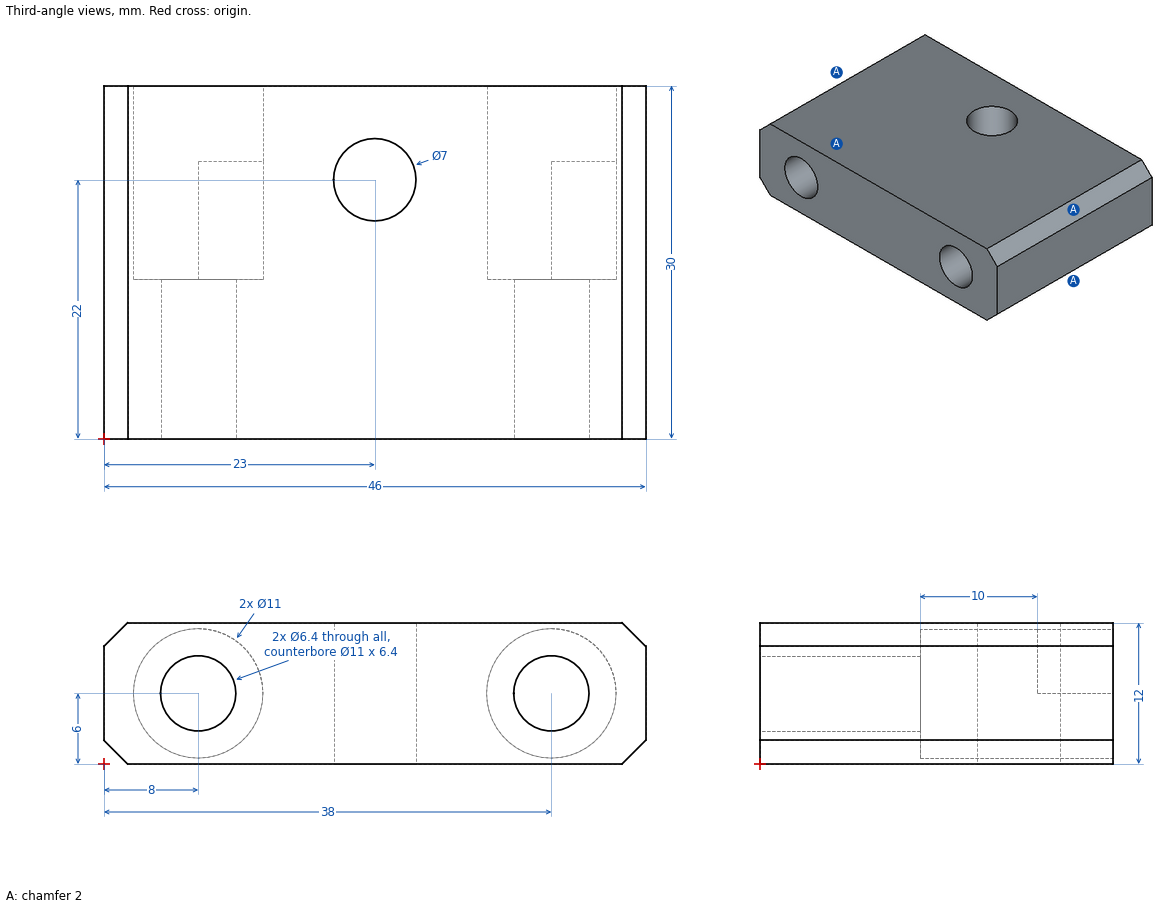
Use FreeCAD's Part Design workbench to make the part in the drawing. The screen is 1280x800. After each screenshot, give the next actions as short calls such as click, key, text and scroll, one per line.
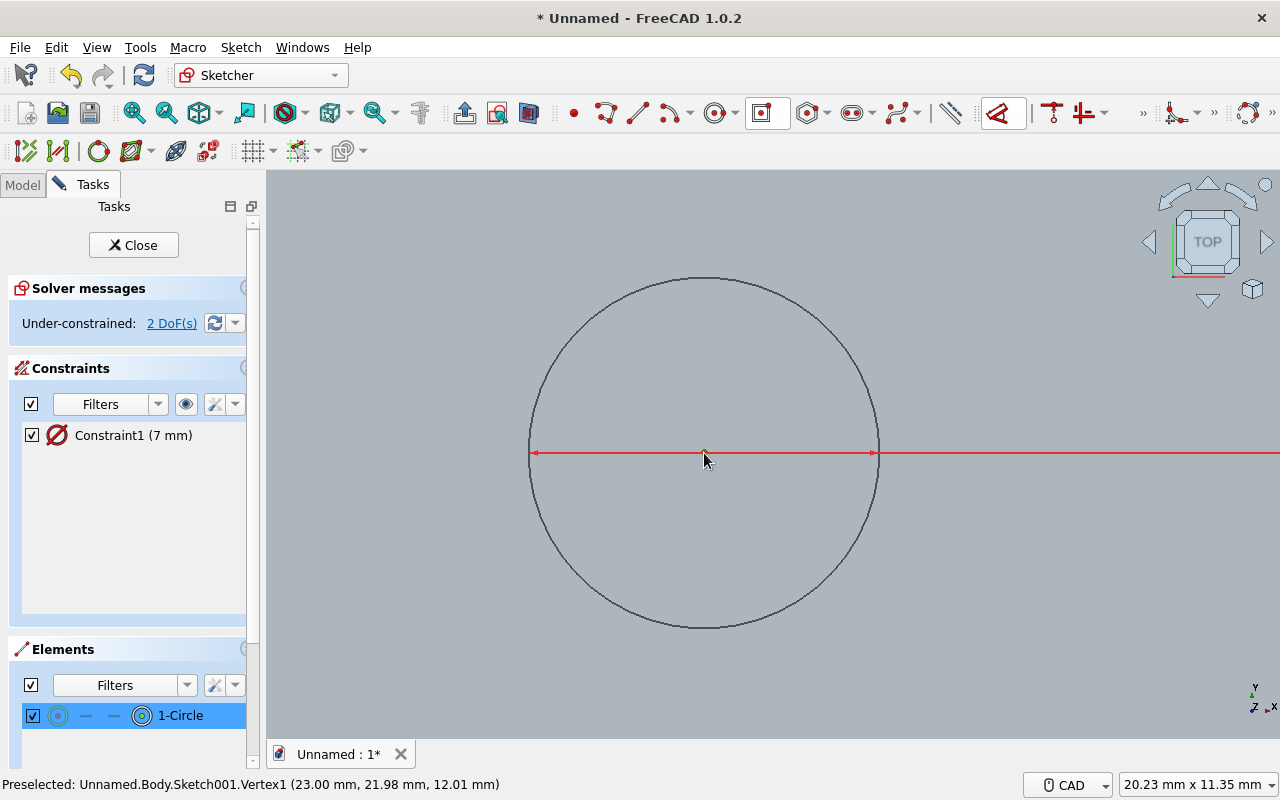
key(l)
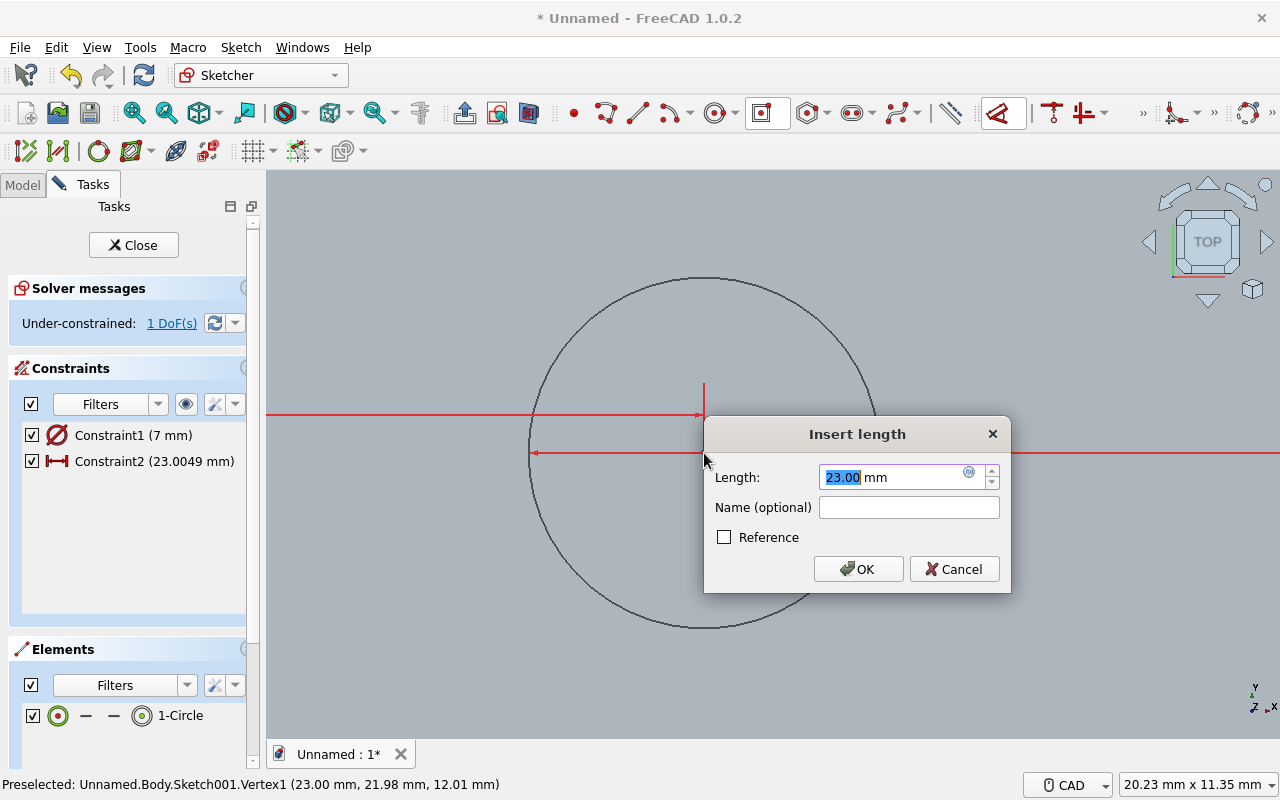
text(23)
key(Return)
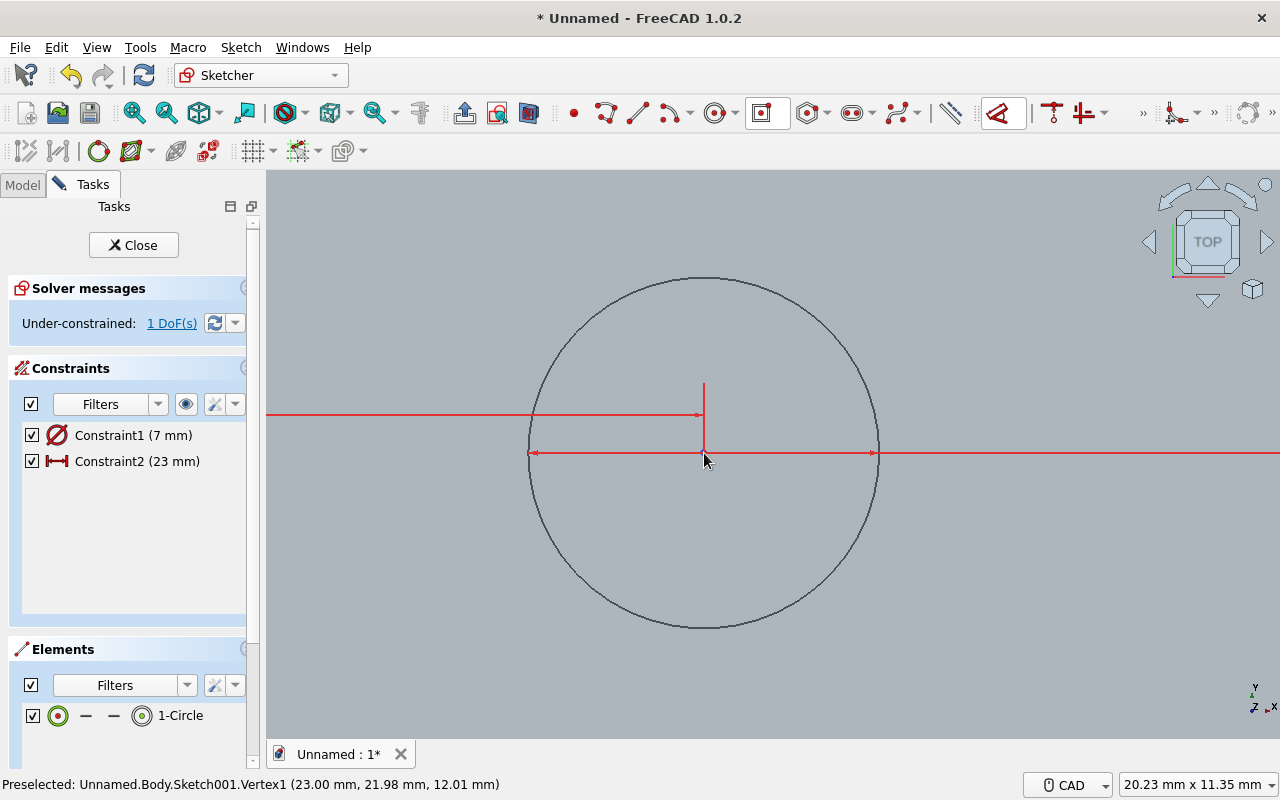
click(704, 453)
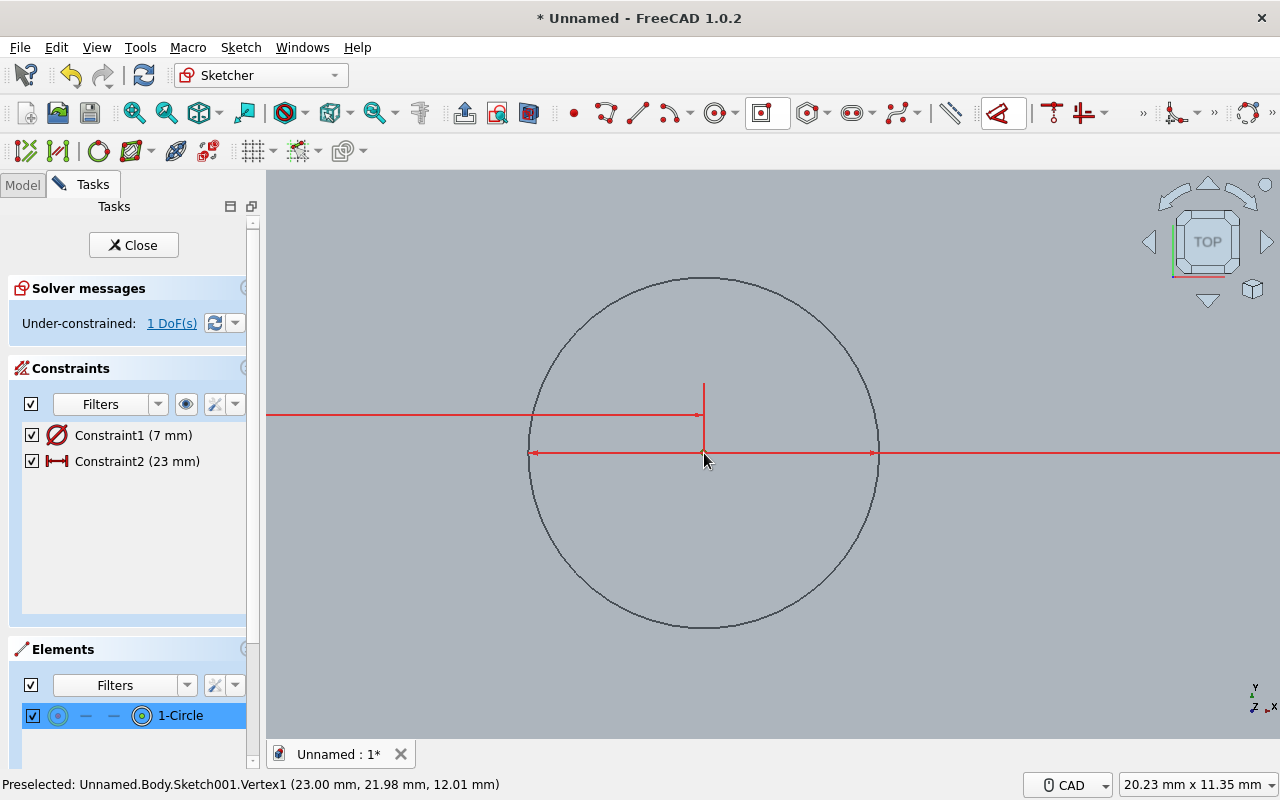
key(i)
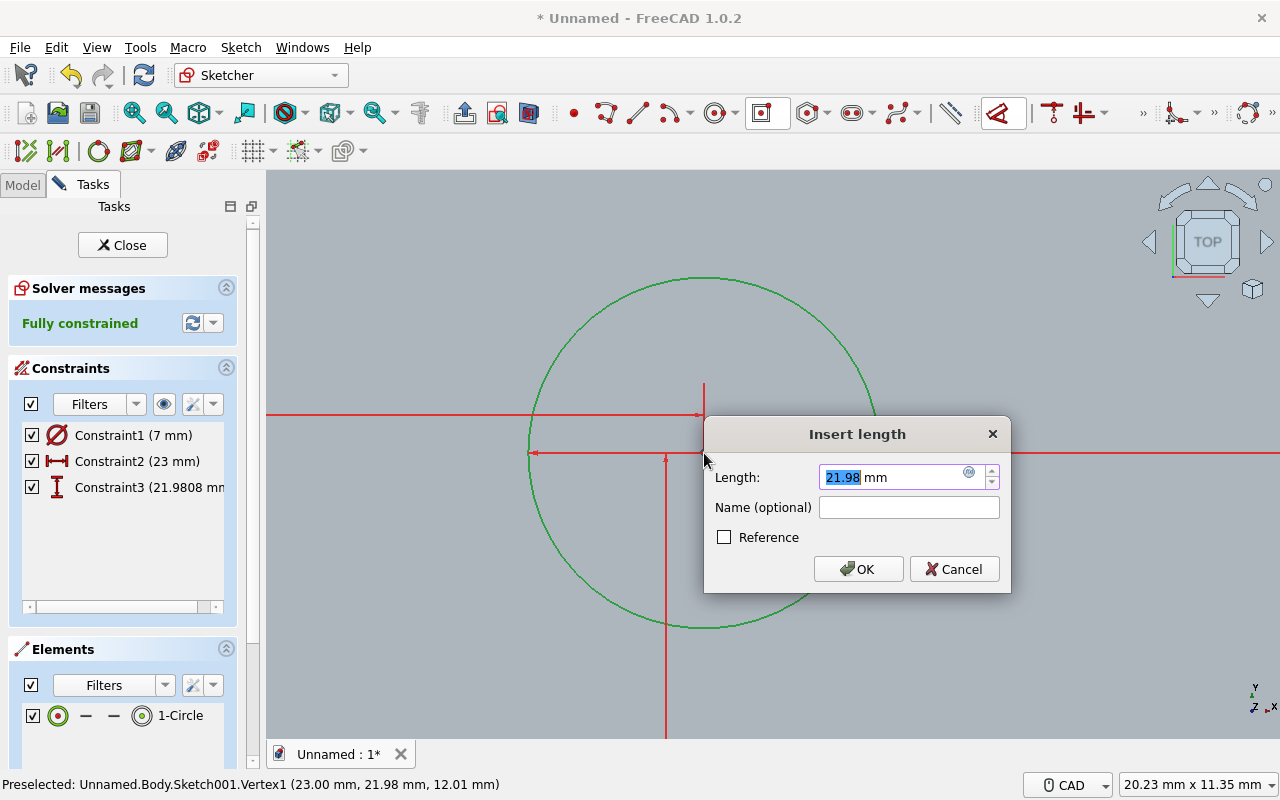
text(22)
key(Return)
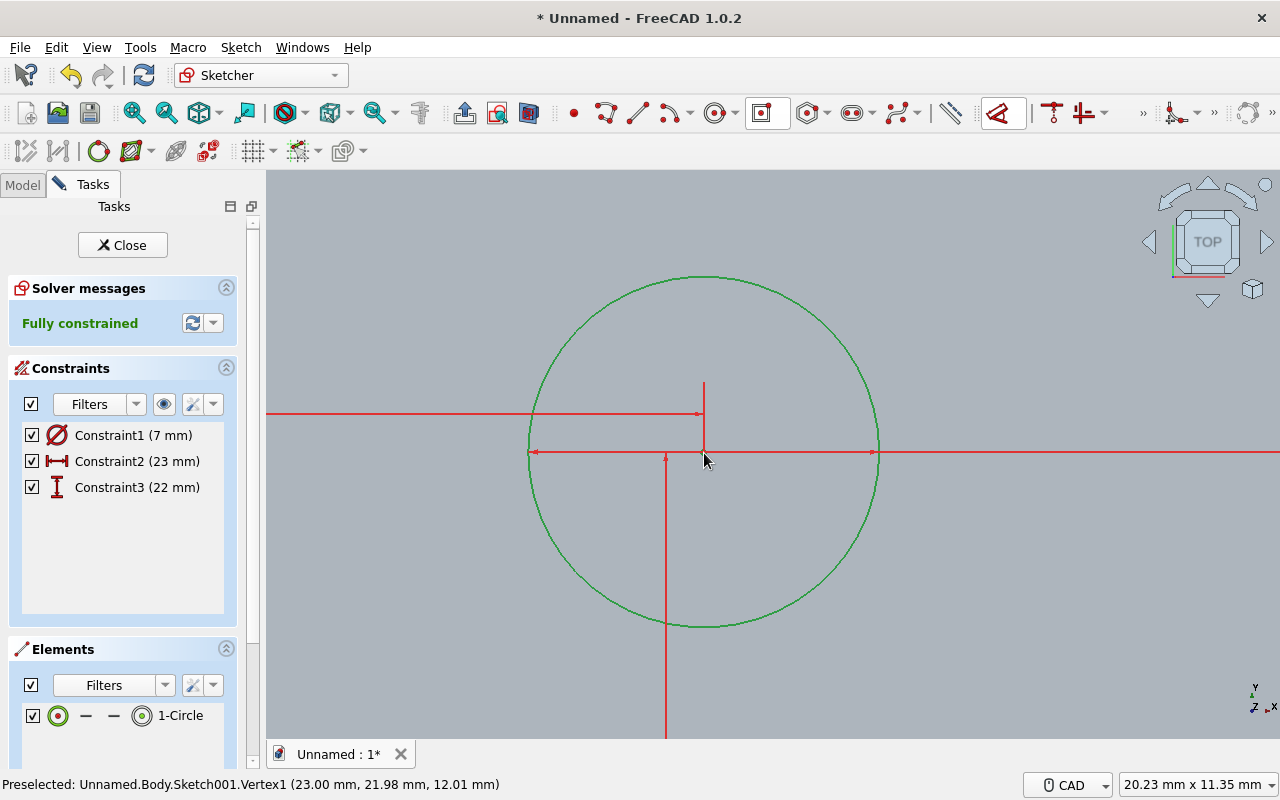
click(123, 245)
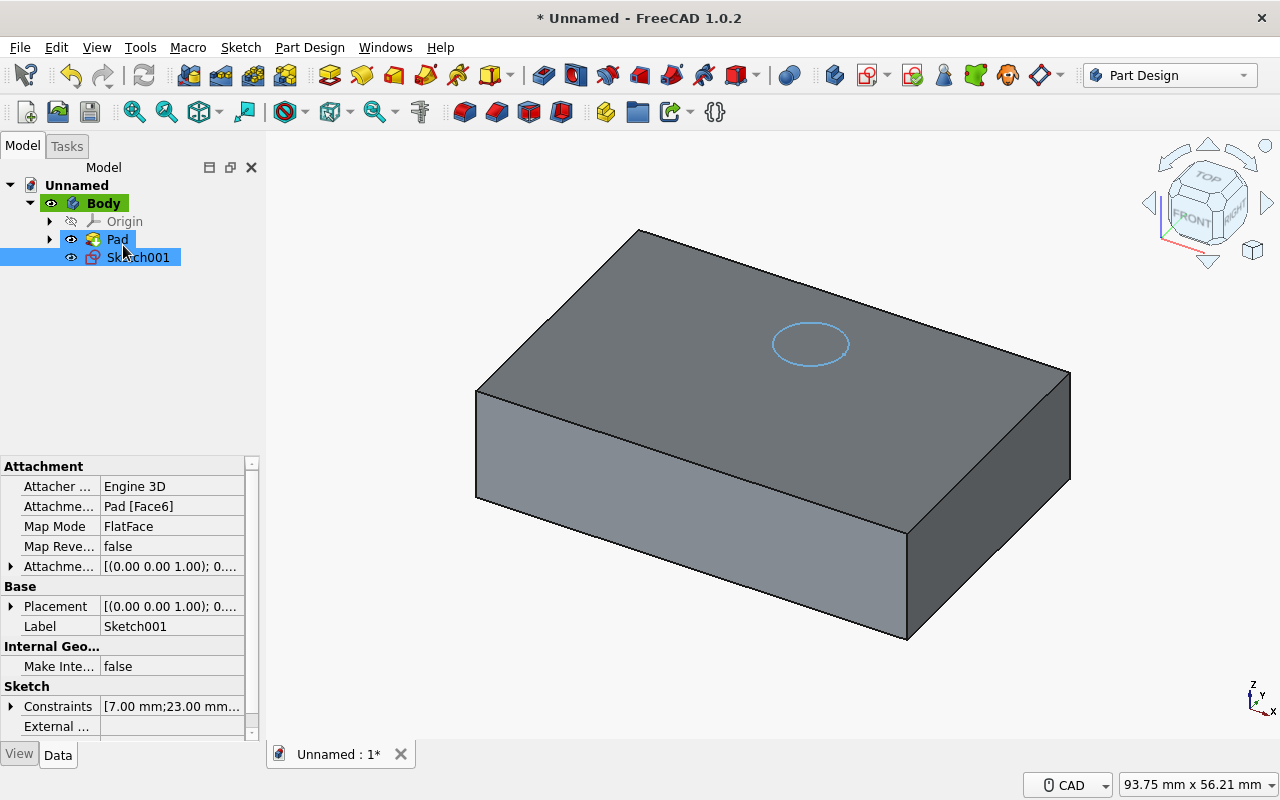
click(544, 76)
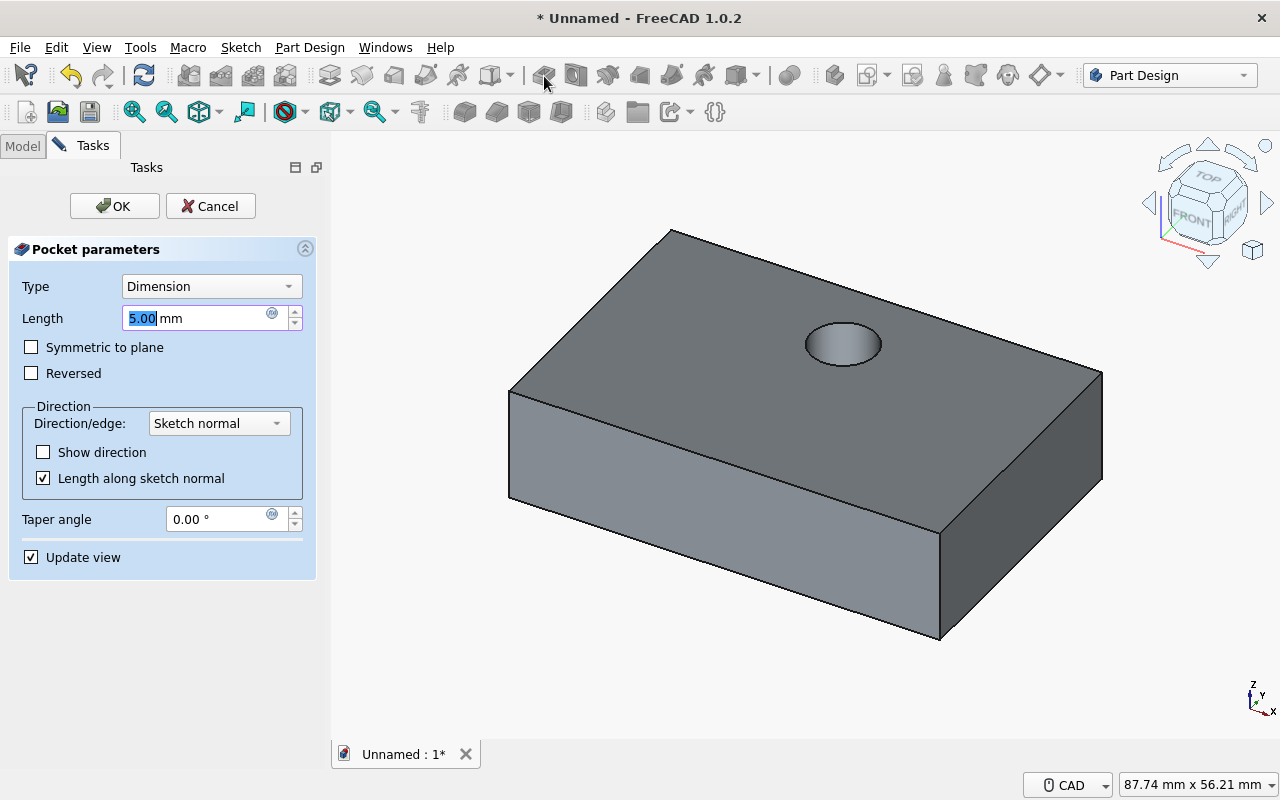
click(212, 286)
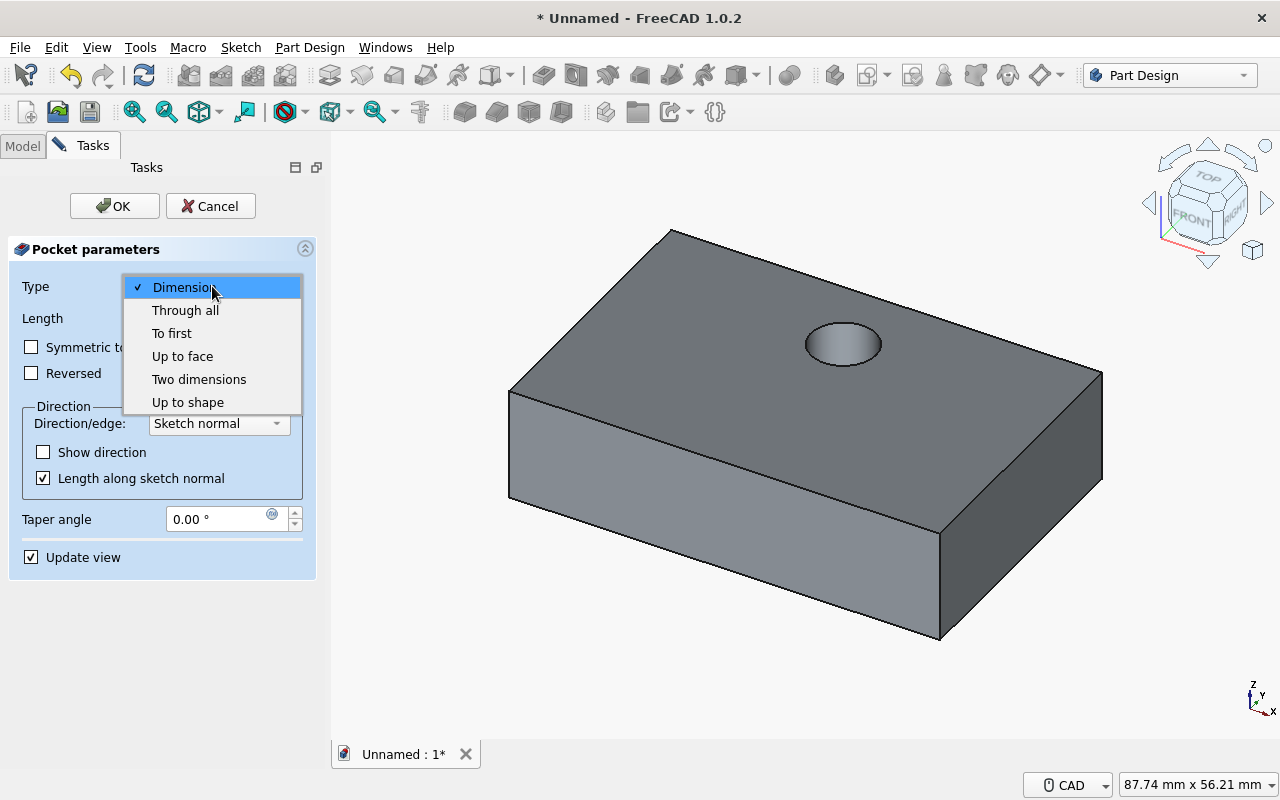
click(212, 310)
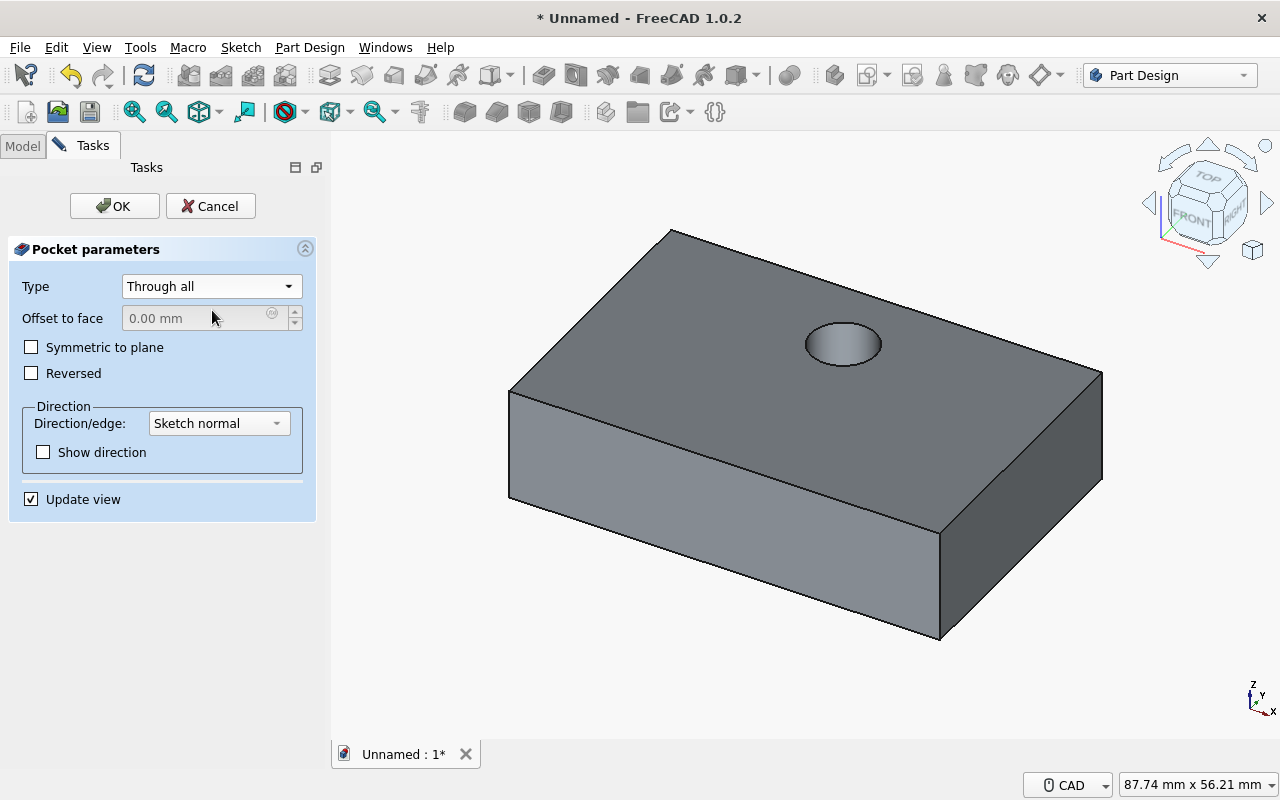
click(115, 206)